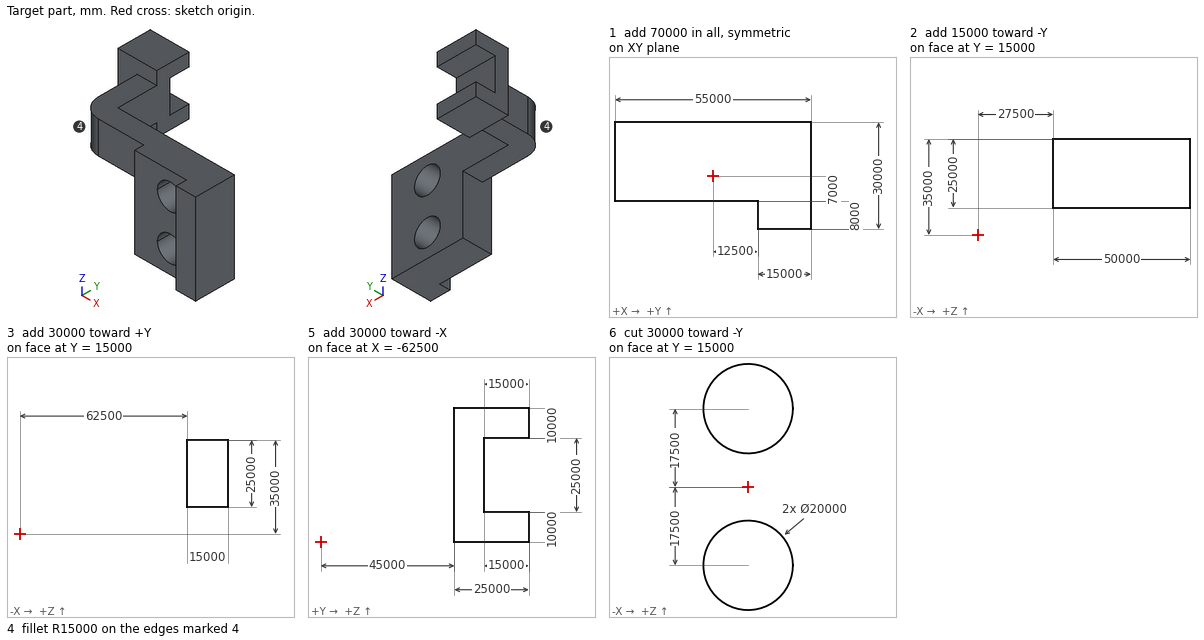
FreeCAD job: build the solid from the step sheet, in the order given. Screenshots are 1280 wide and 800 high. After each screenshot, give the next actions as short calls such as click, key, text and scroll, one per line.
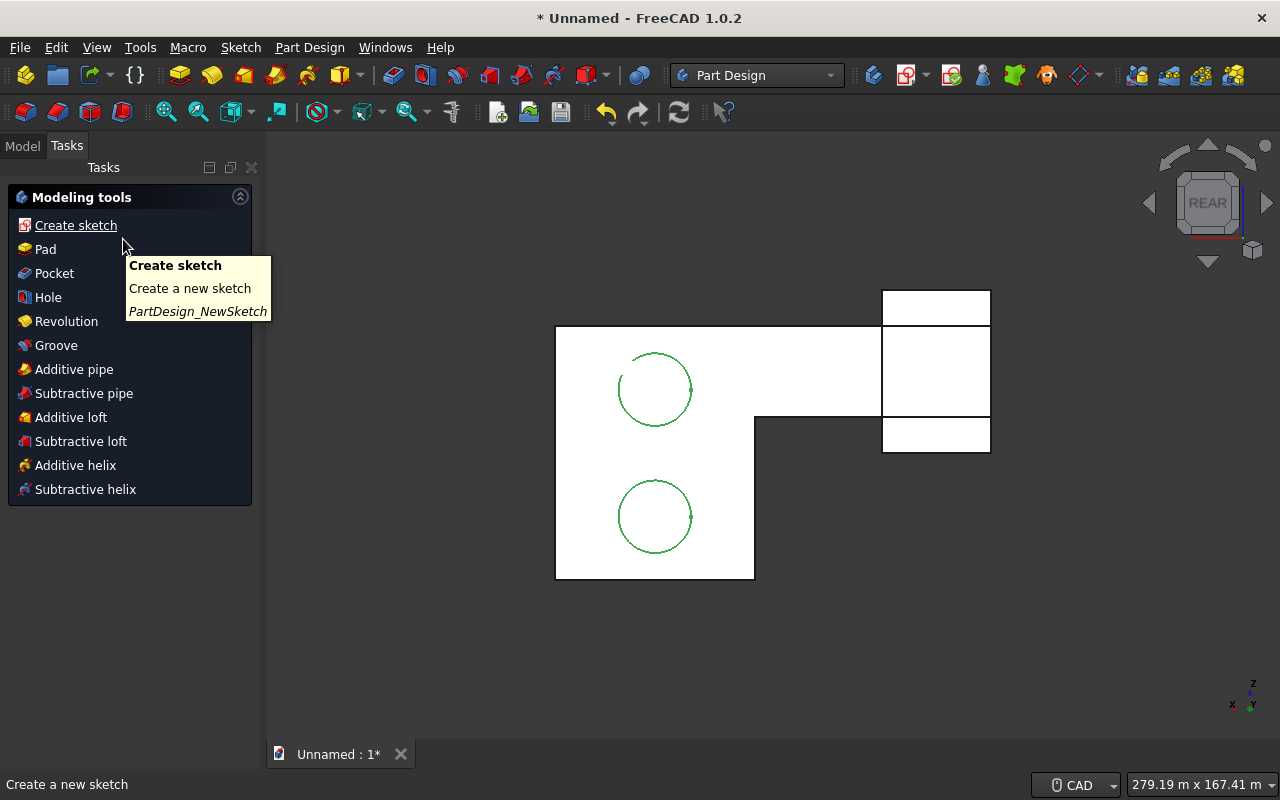
click(394, 76)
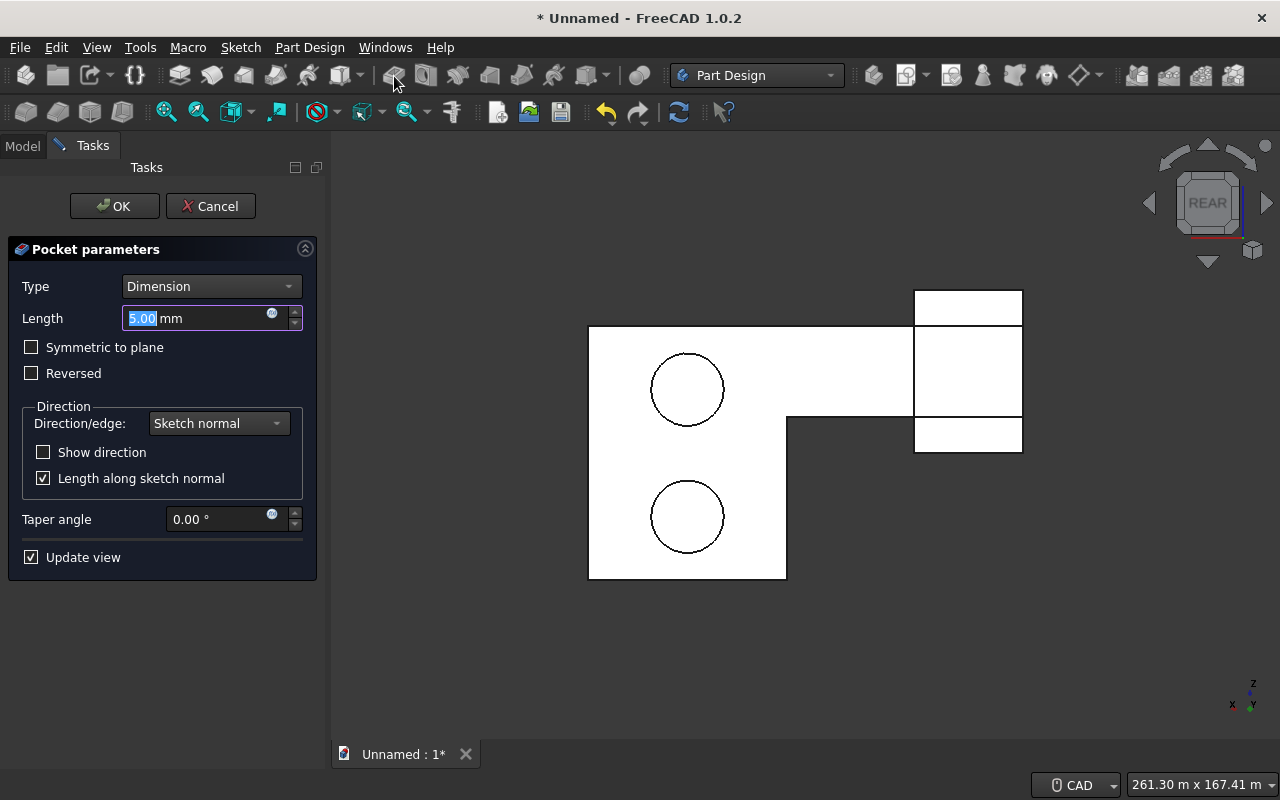
text(30000)
key(Tab)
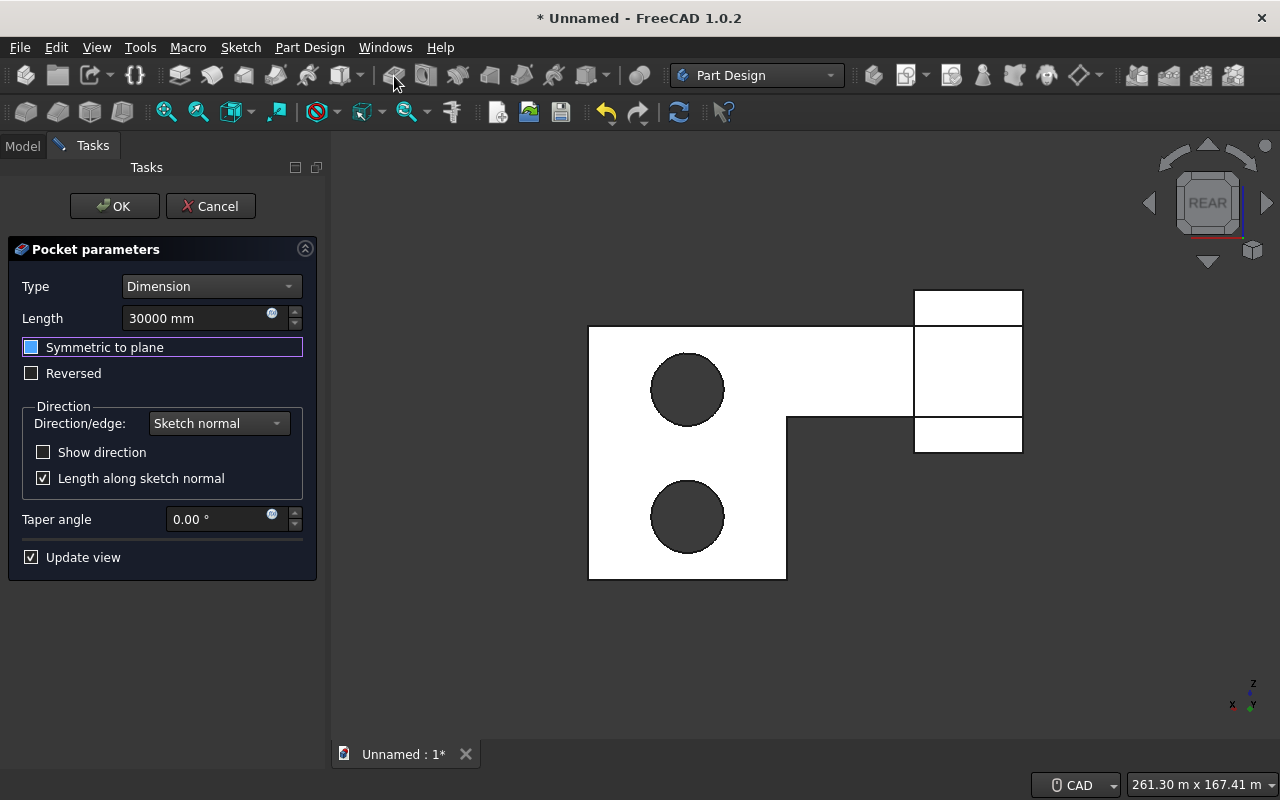
click(115, 206)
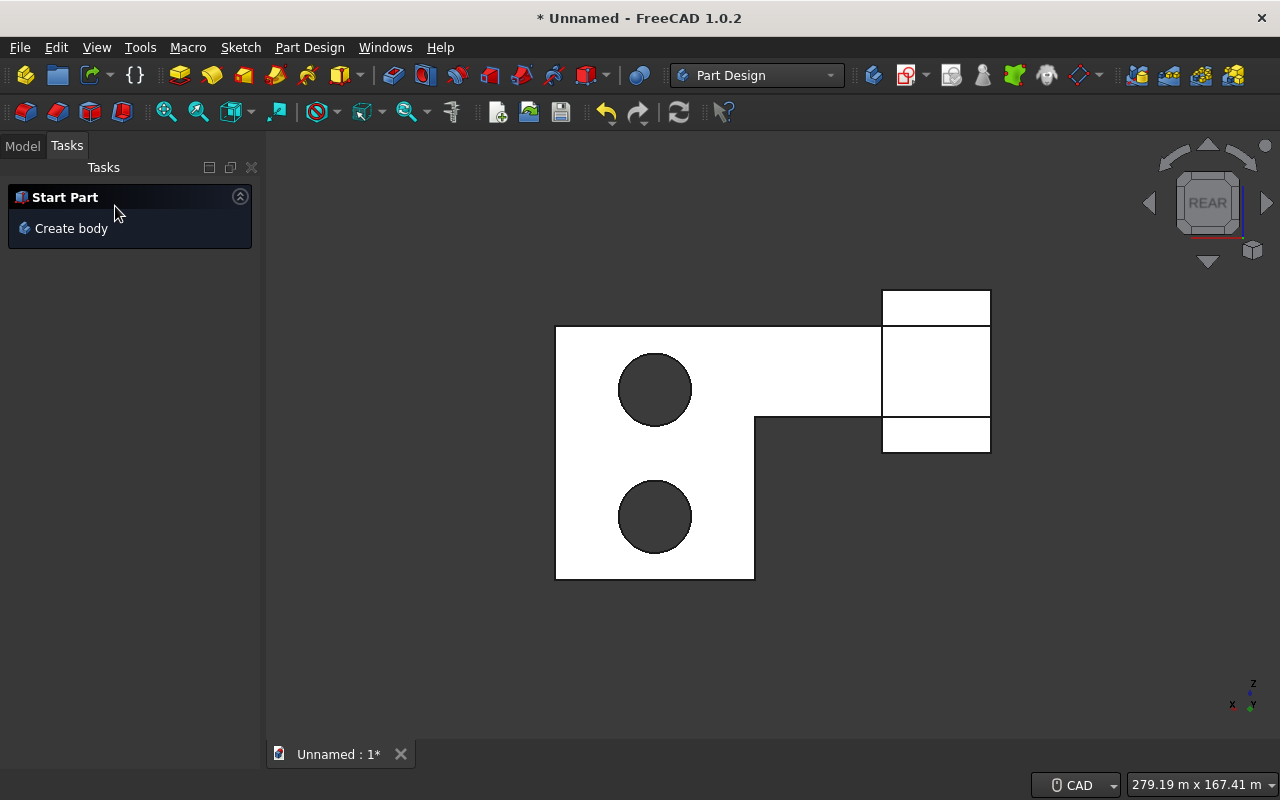
key(0)